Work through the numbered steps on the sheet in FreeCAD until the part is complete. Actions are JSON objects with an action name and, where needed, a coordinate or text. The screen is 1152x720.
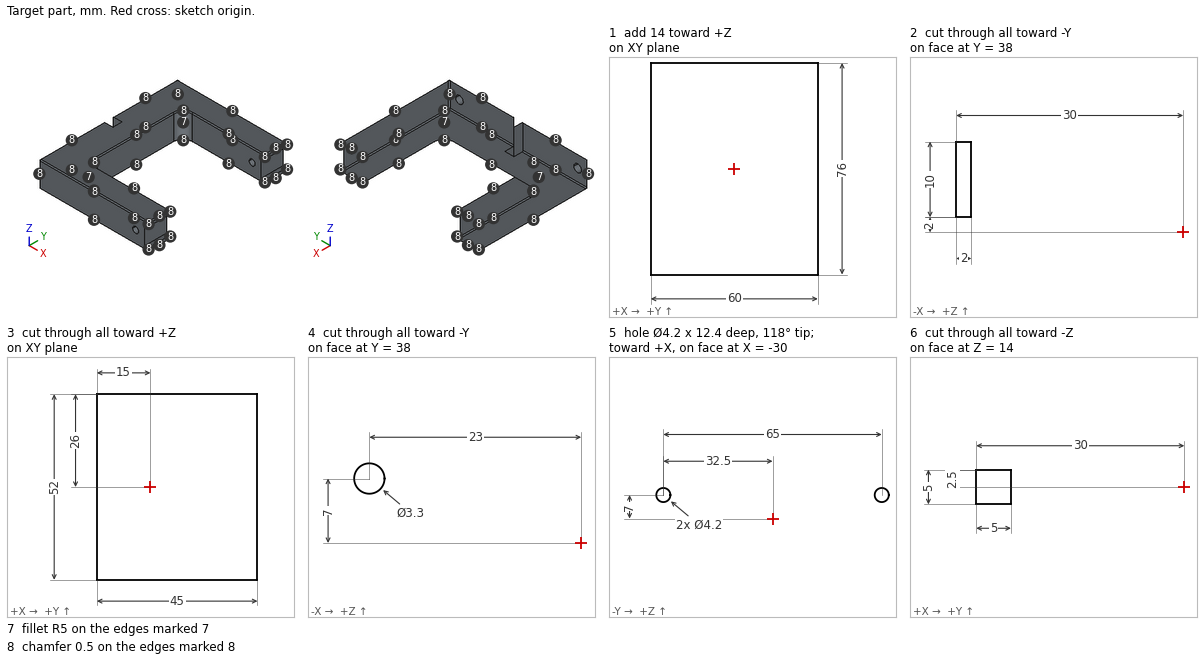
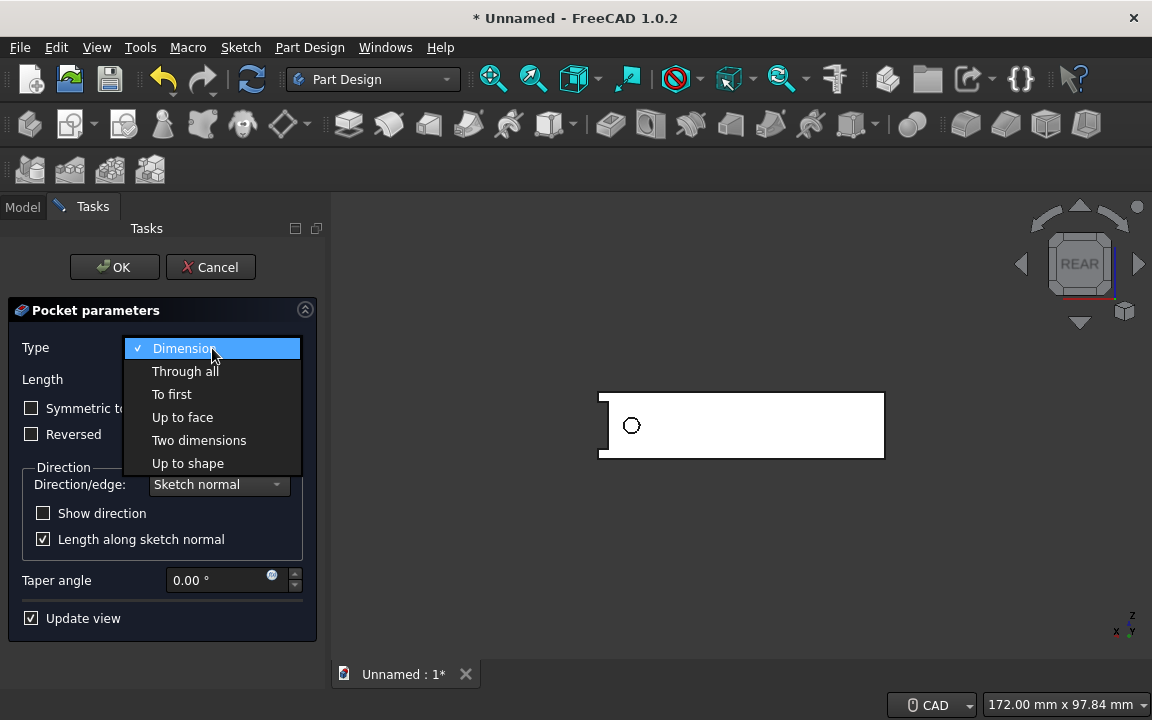
{"action": "left_click", "coordinate": [212, 372]}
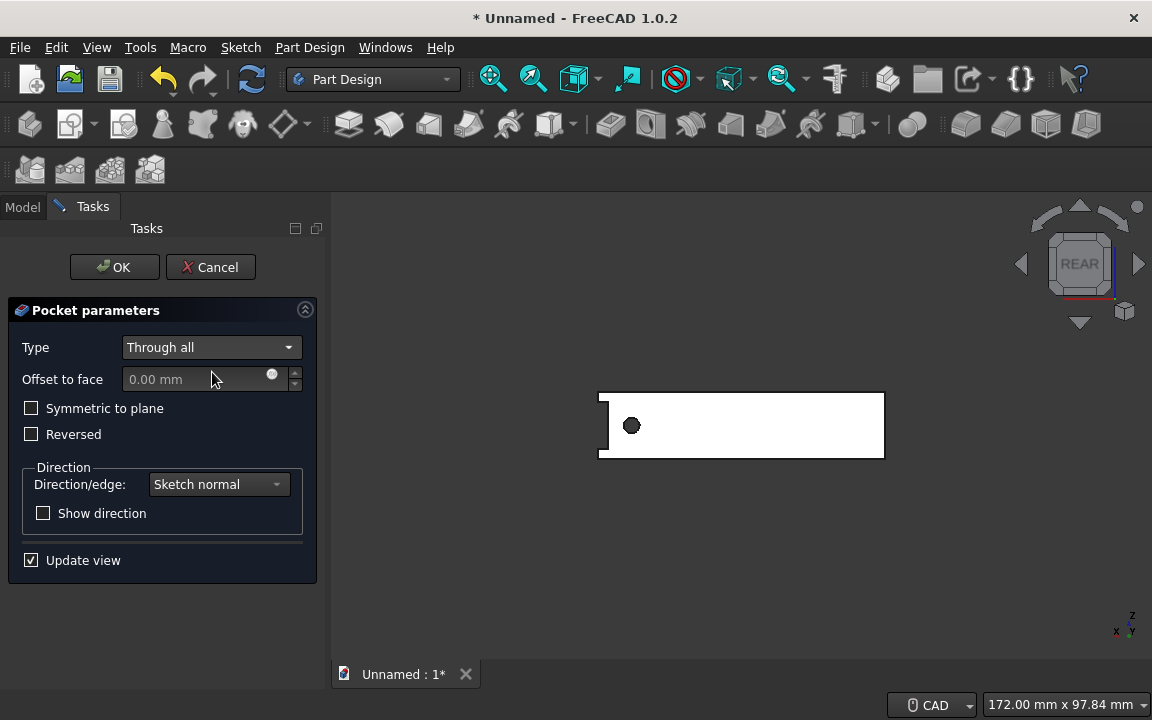
{"action": "left_click", "coordinate": [115, 267]}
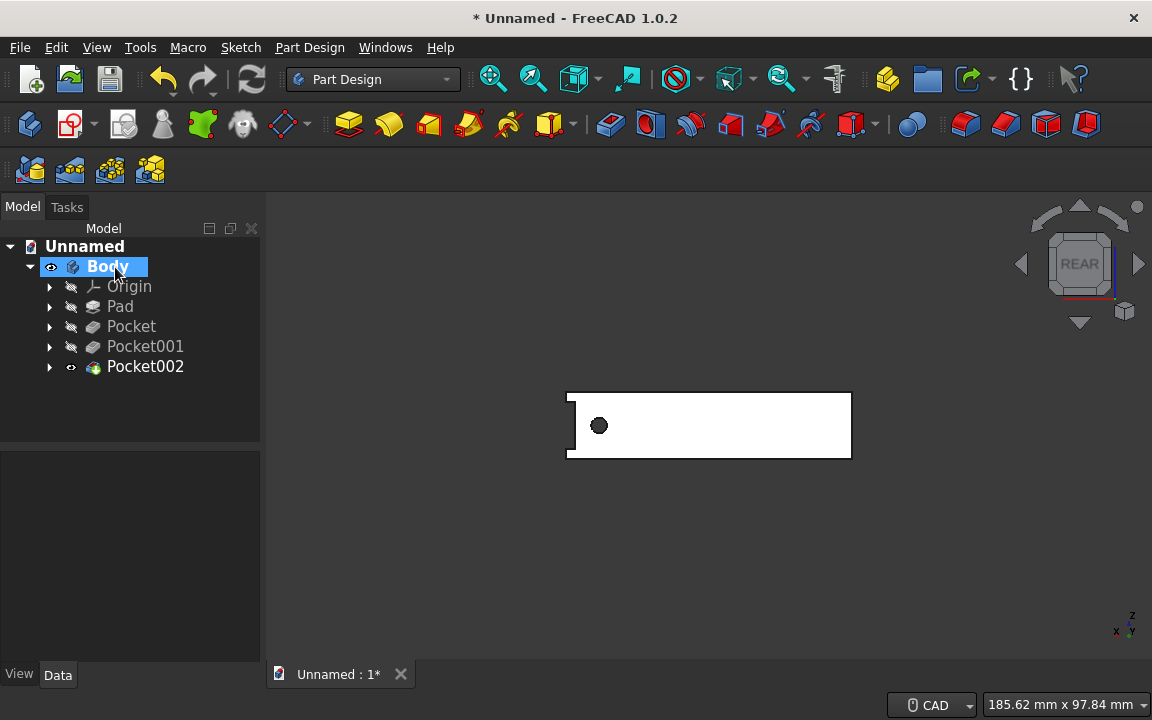
{"action": "left_click", "coordinate": [494, 80]}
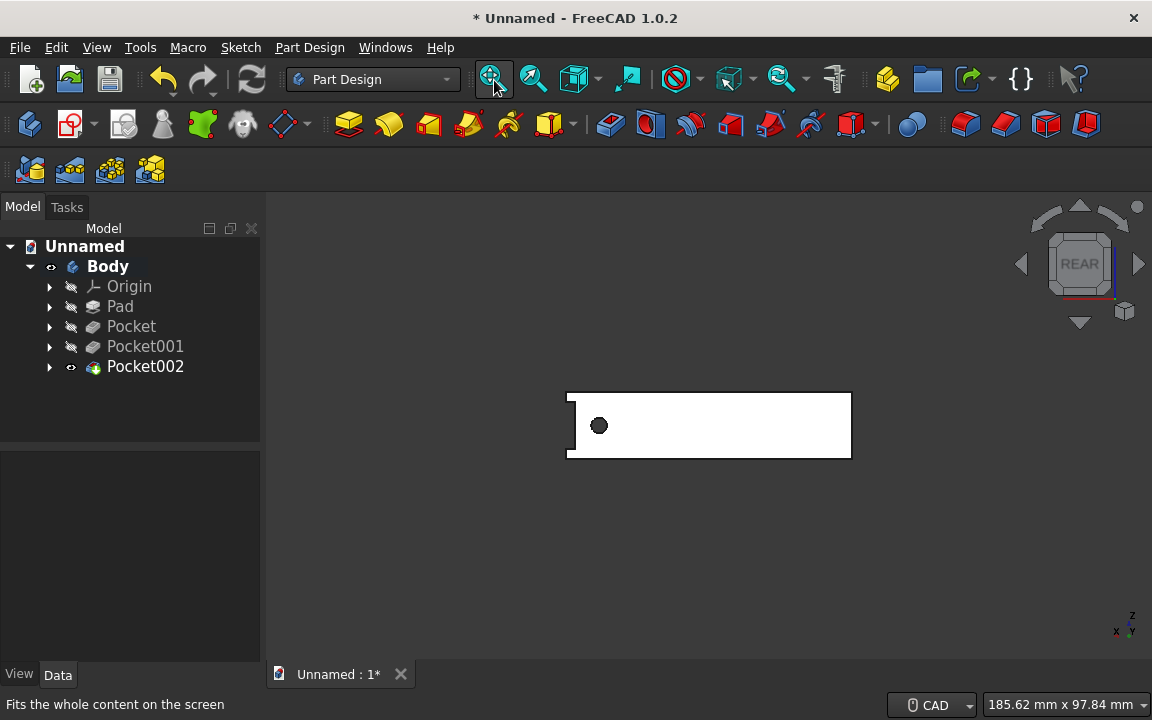
{"action": "key", "text": "6"}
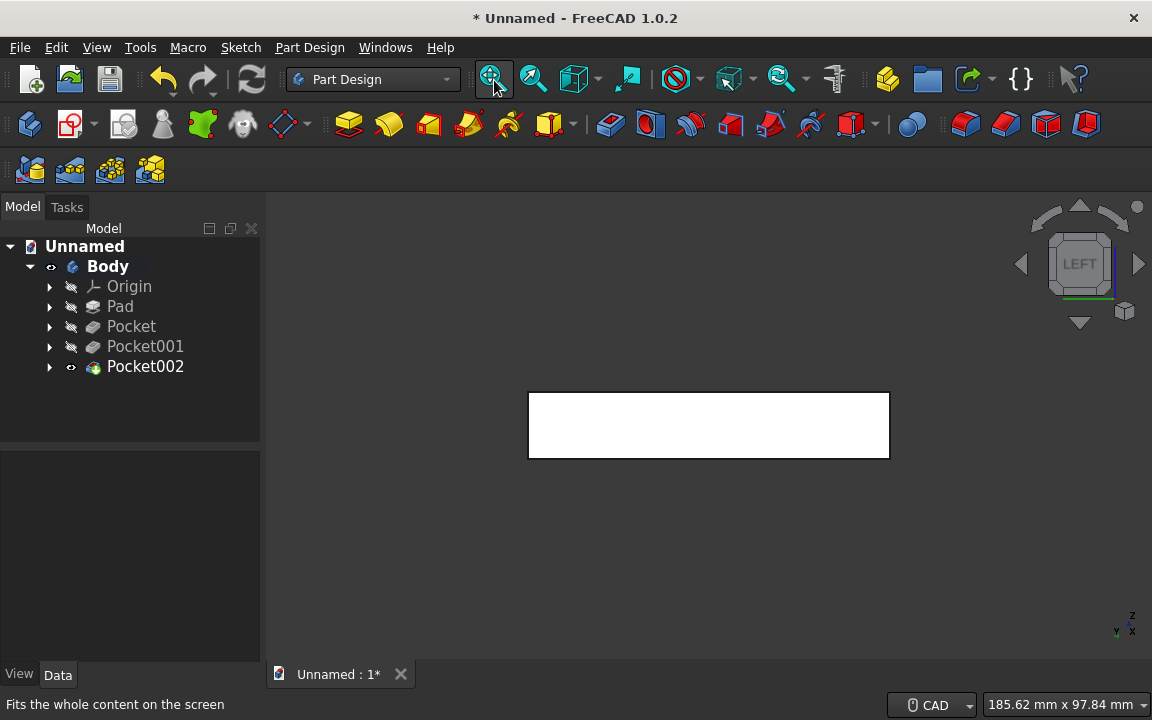
{"action": "key", "text": "v f"}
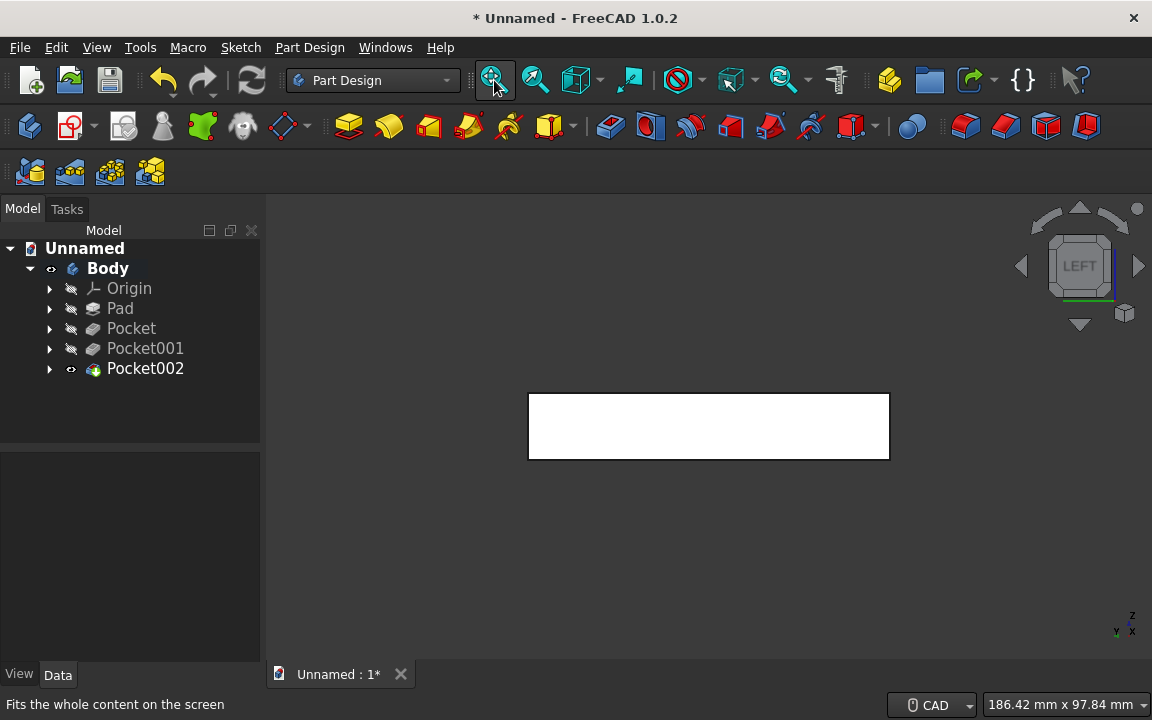
{"action": "left_click", "coordinate": [606, 425]}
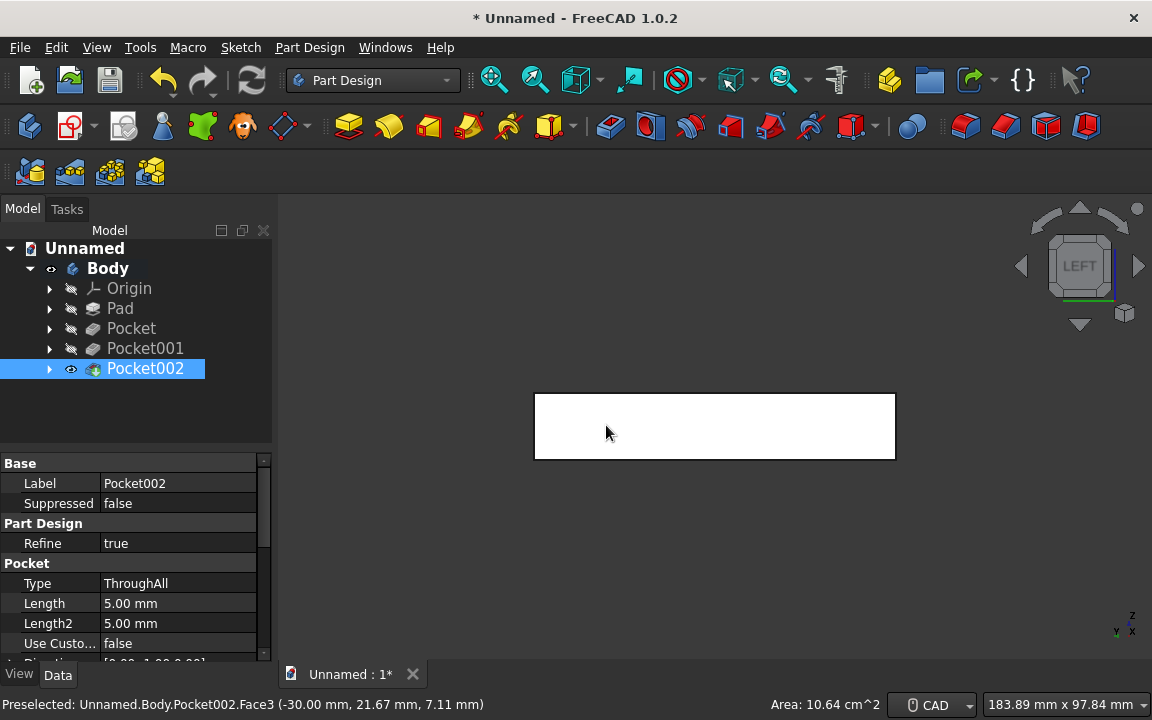
{"action": "left_click", "coordinate": [70, 126]}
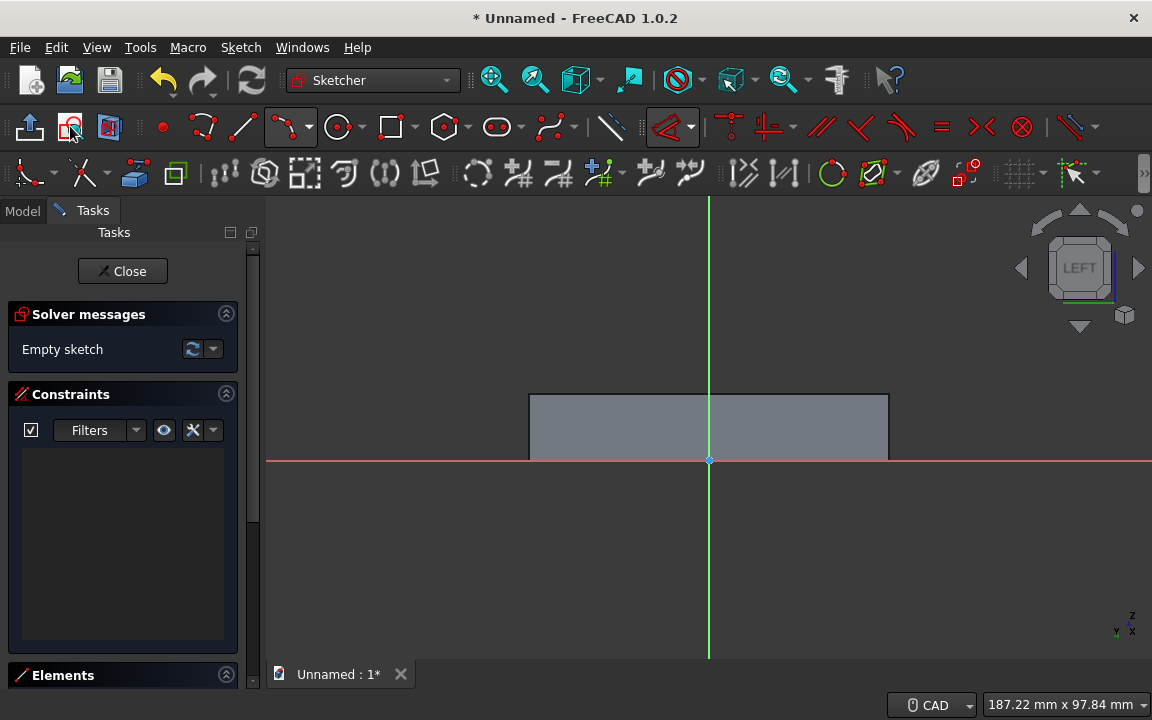
{"action": "scroll", "coordinate": [848, 463], "scroll_direction": "up", "scroll_amount": 2}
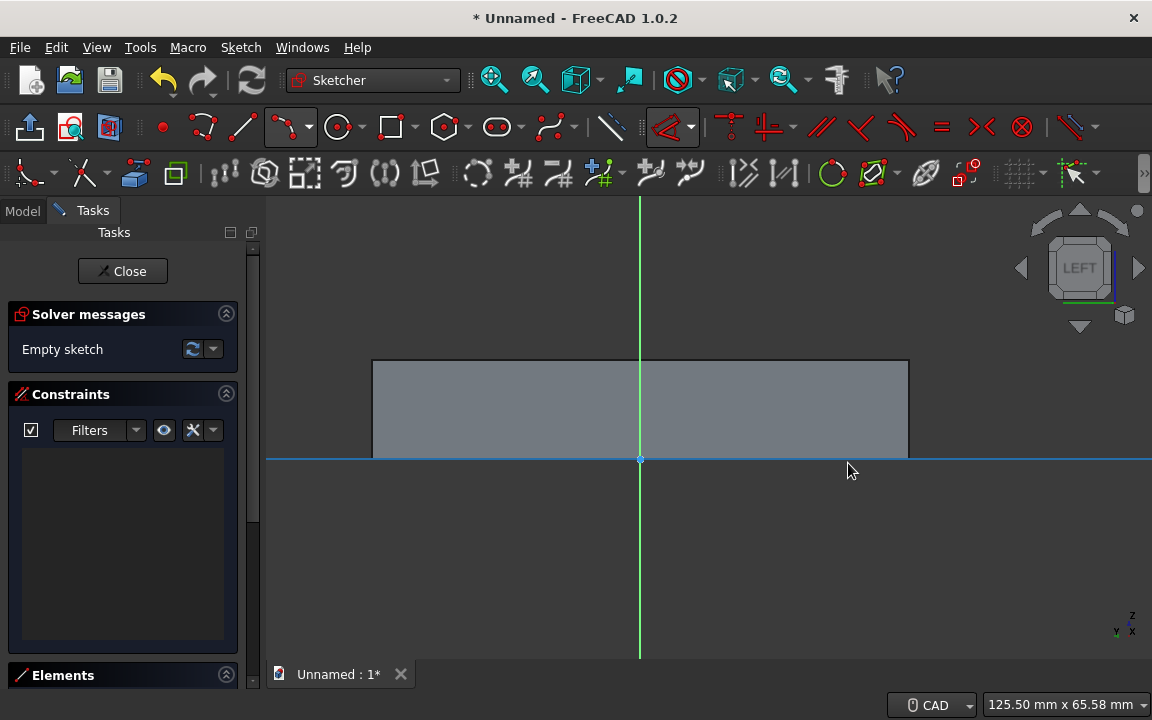
{"action": "key", "text": "g c"}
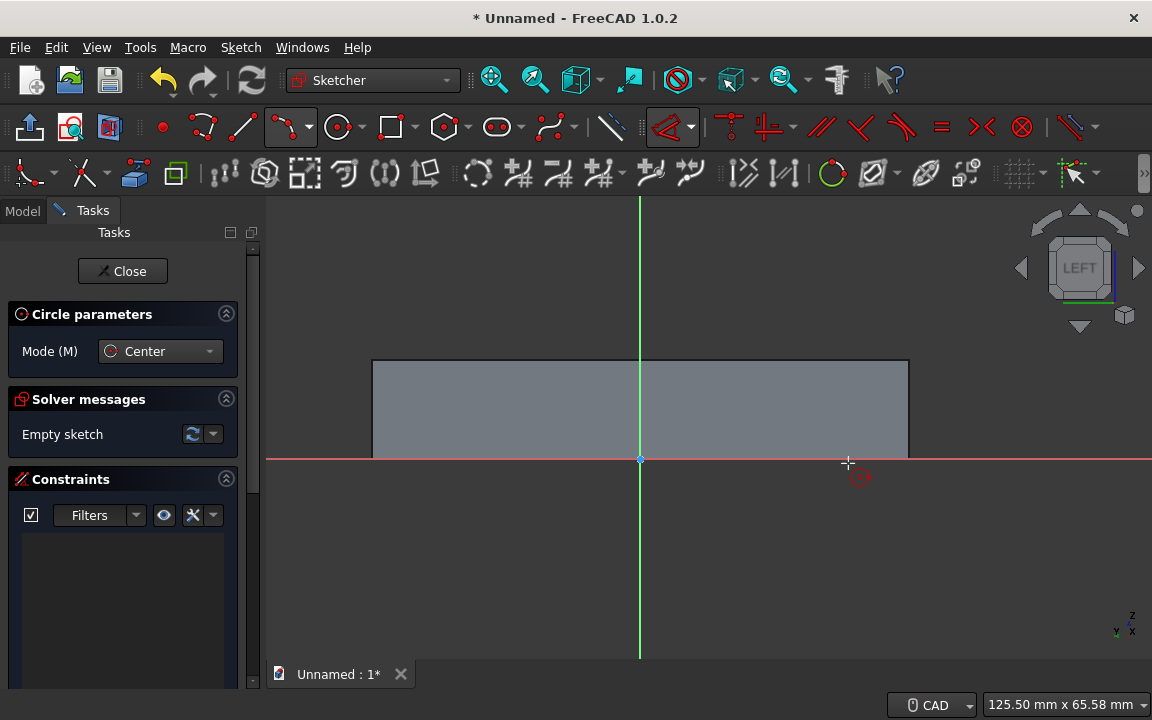
{"action": "scroll", "coordinate": [411, 410], "scroll_direction": "up", "scroll_amount": 3}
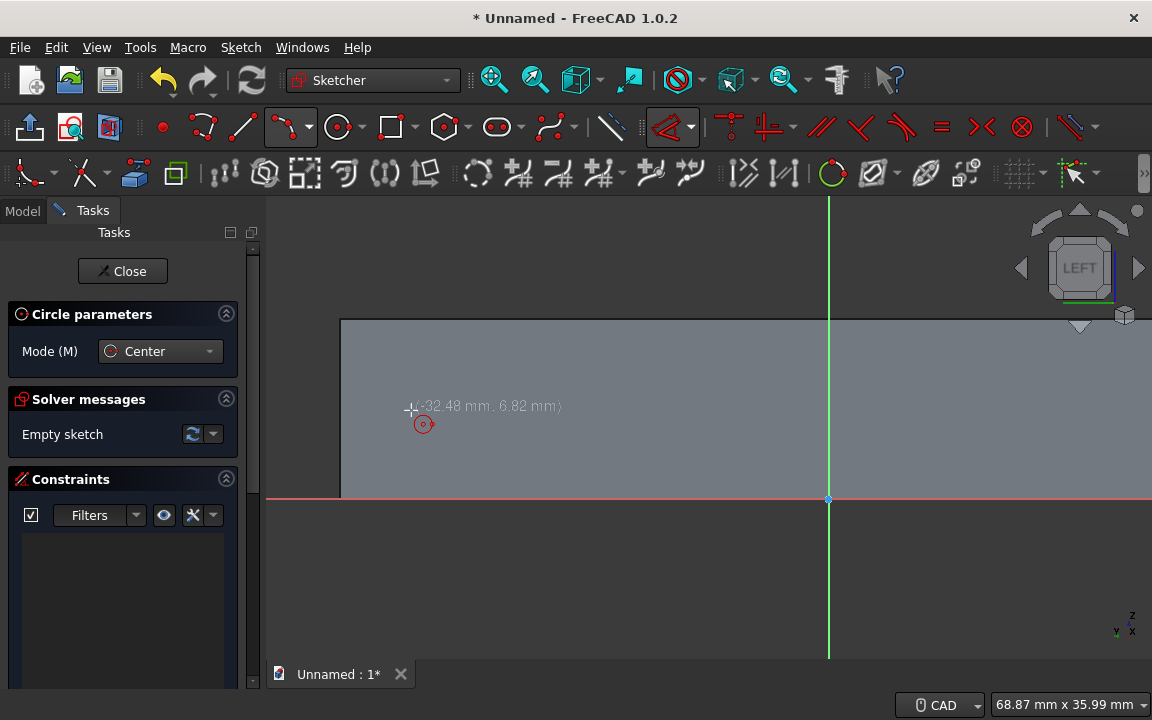
{"action": "left_click", "coordinate": [411, 409]}
{"action": "left_click", "coordinate": [430, 390]}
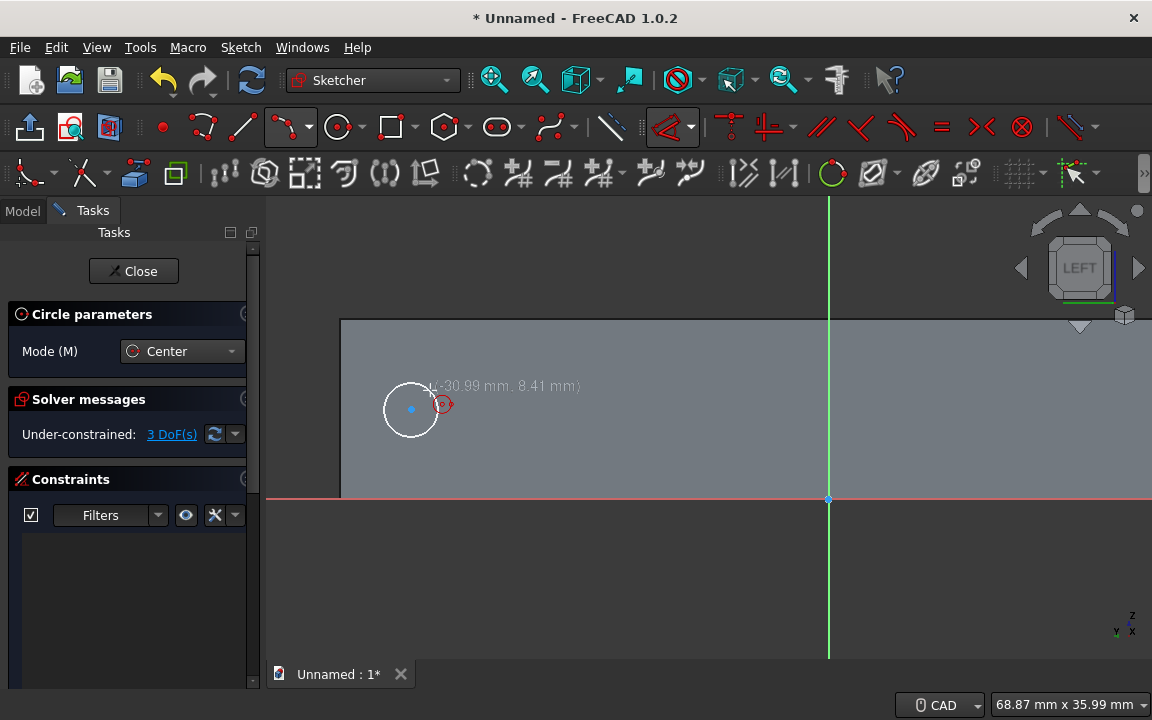
{"action": "scroll", "coordinate": [412, 411], "scroll_direction": "down", "scroll_amount": 3}